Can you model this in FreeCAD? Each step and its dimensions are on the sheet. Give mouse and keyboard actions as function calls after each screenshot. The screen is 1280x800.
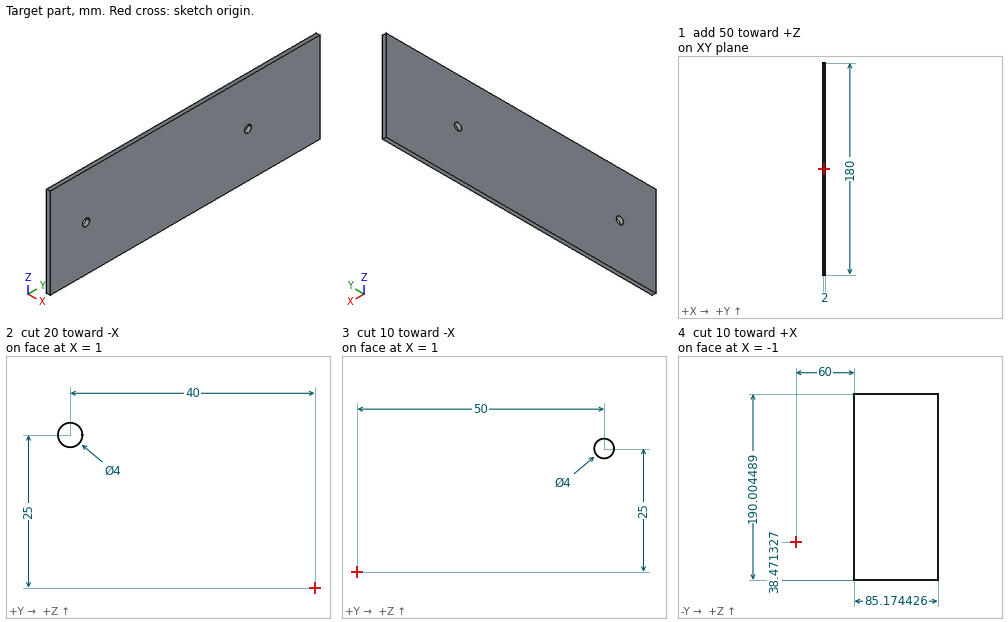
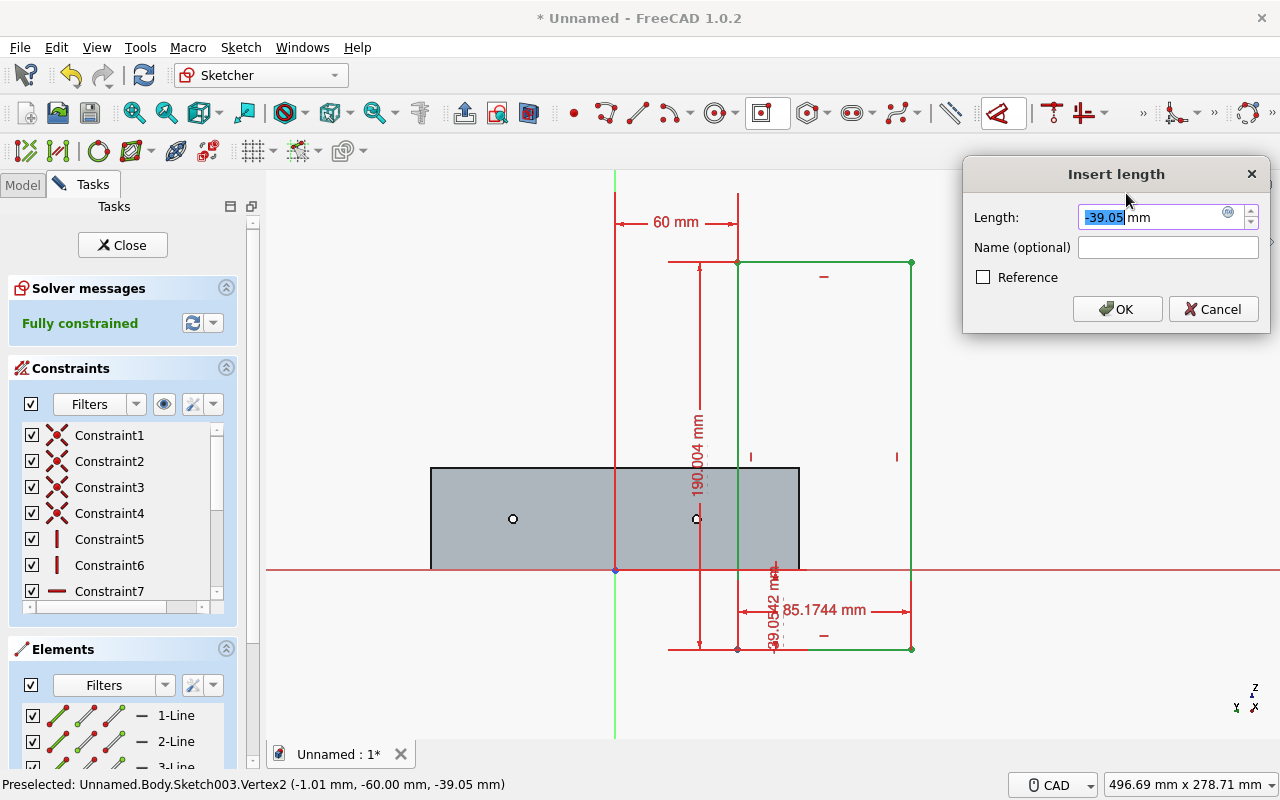
text(-38.471327)
key(Return)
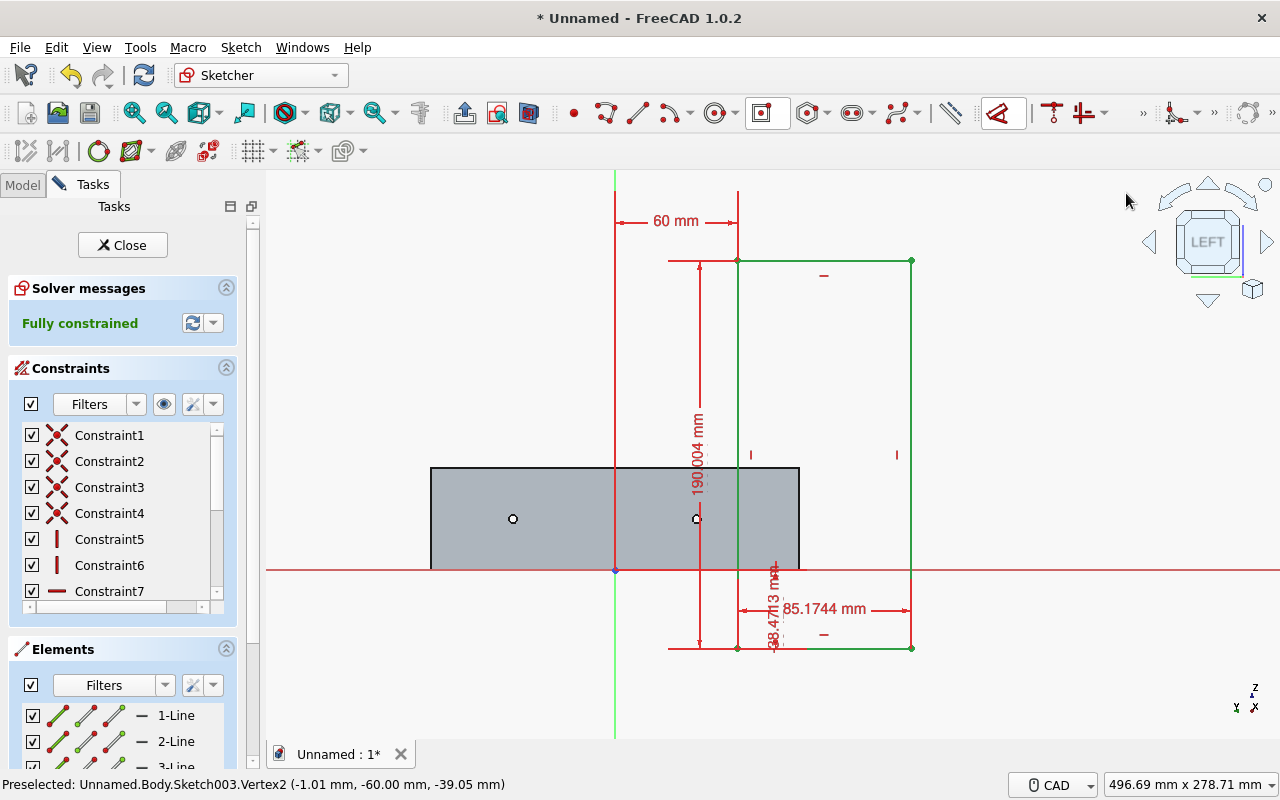
click(123, 245)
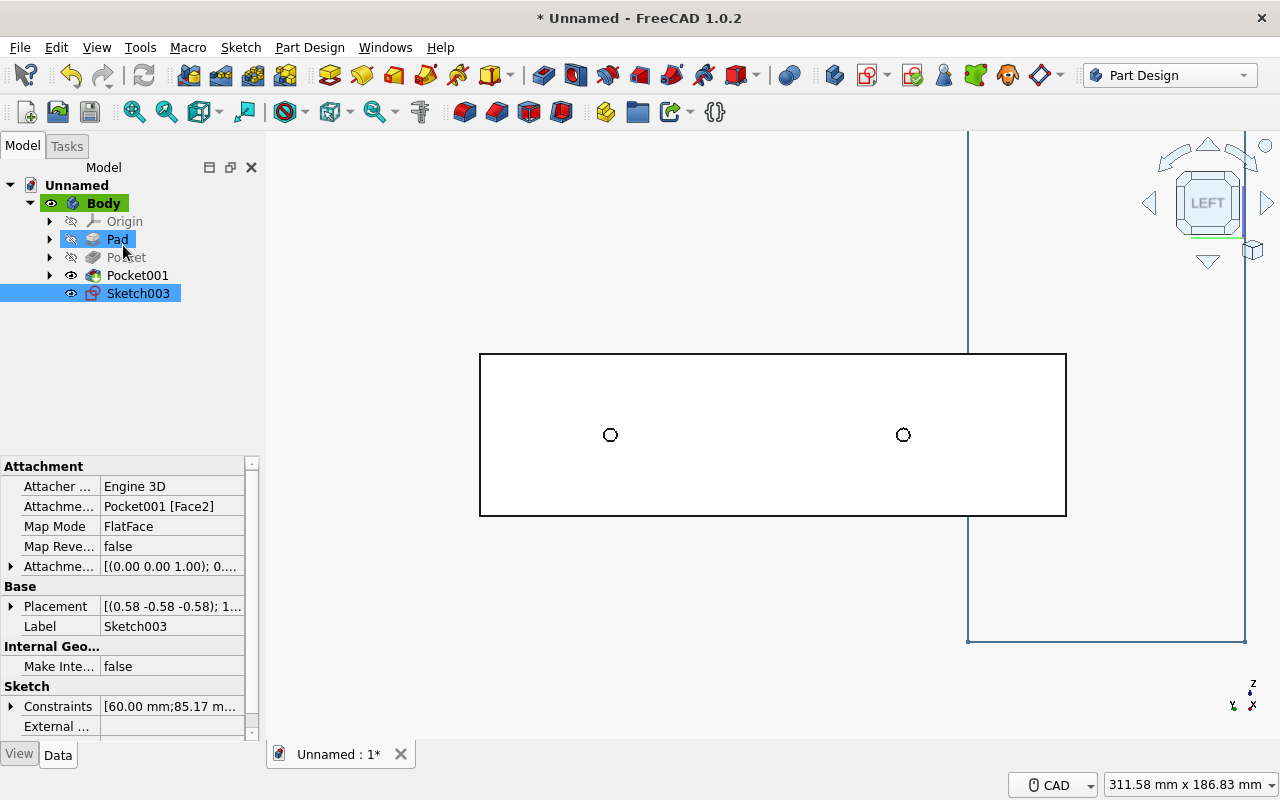
click(544, 76)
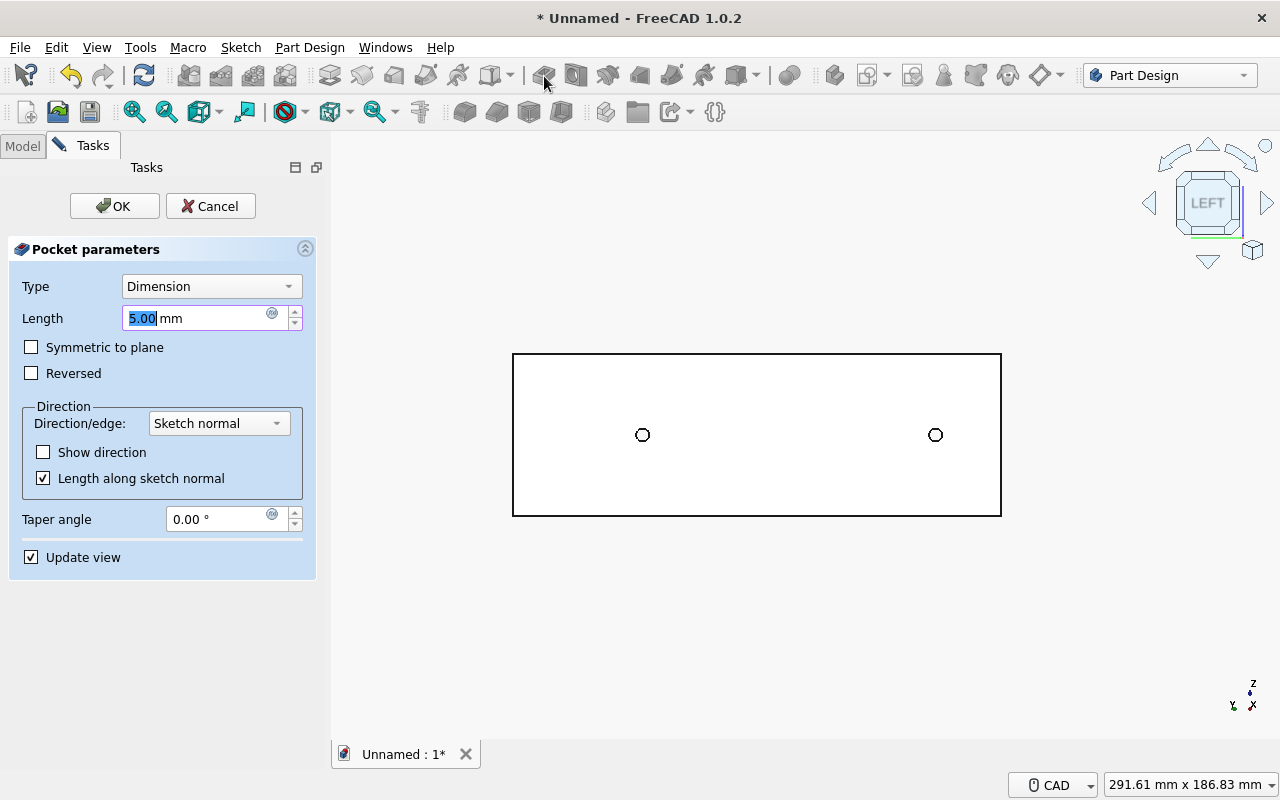
text(10)
key(Tab)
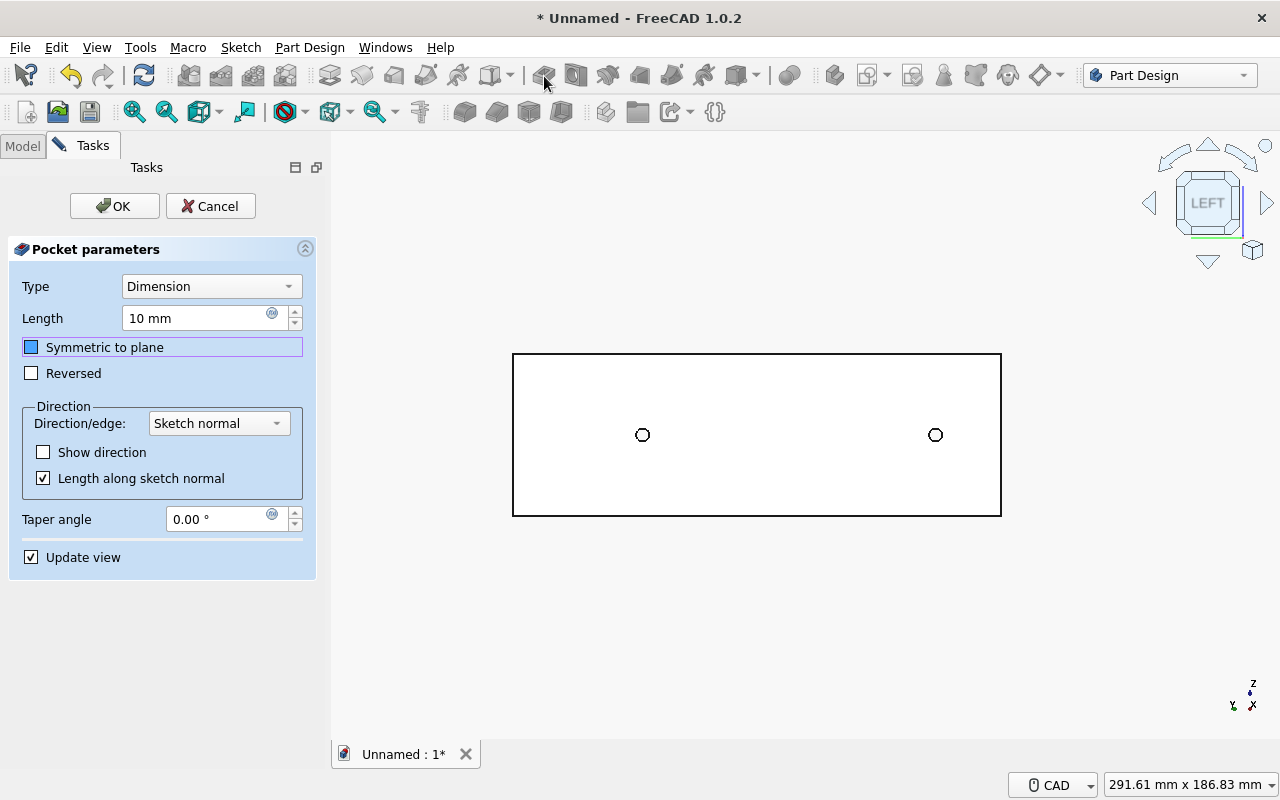
click(115, 206)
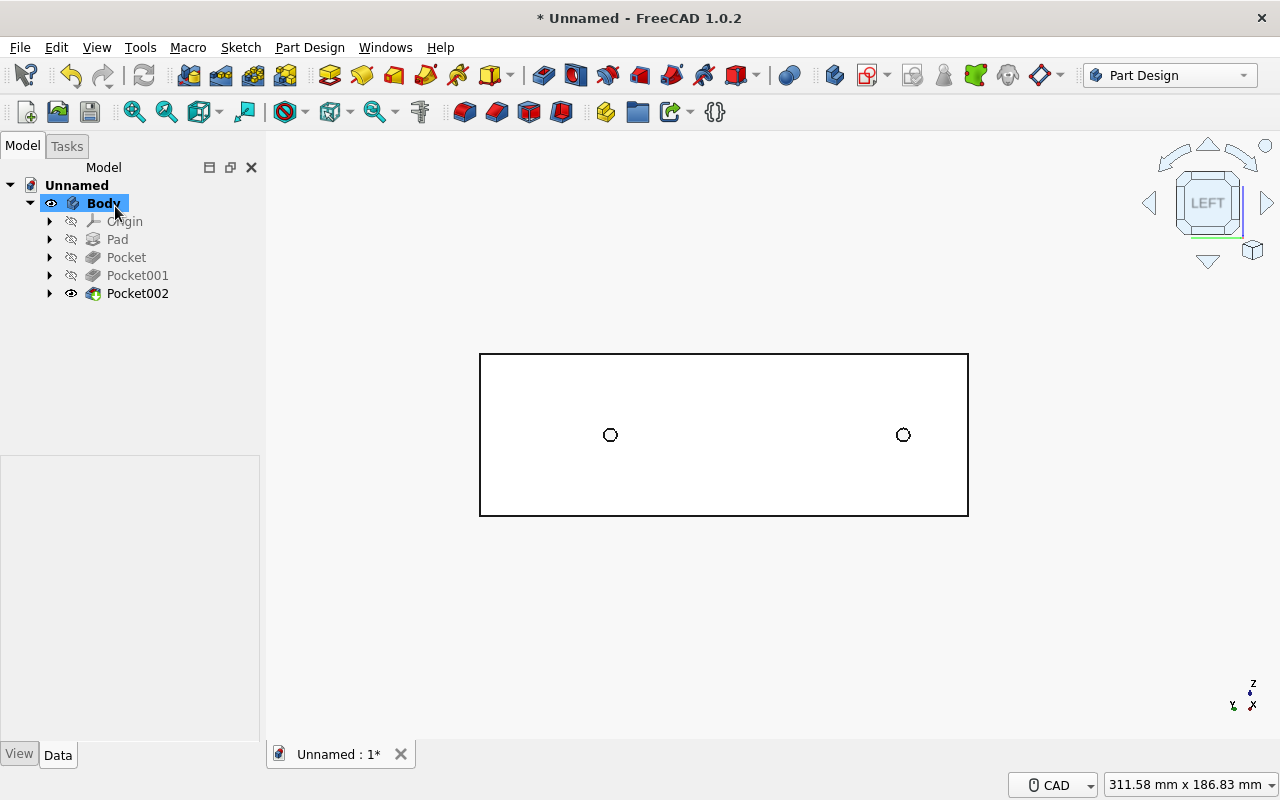
key(0)